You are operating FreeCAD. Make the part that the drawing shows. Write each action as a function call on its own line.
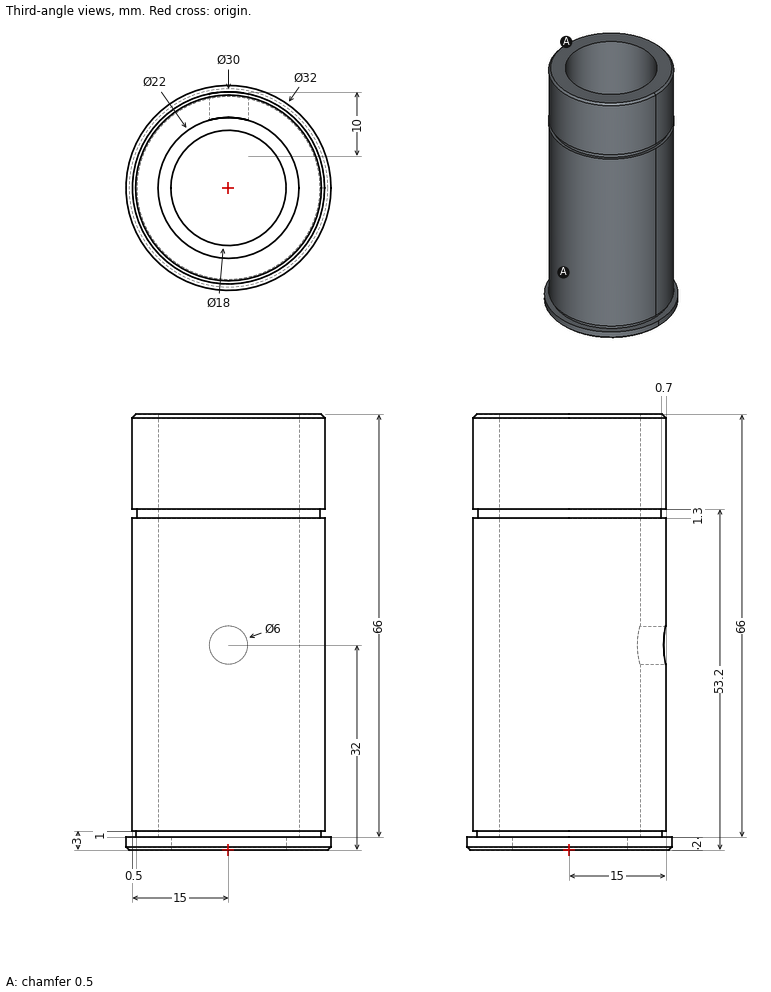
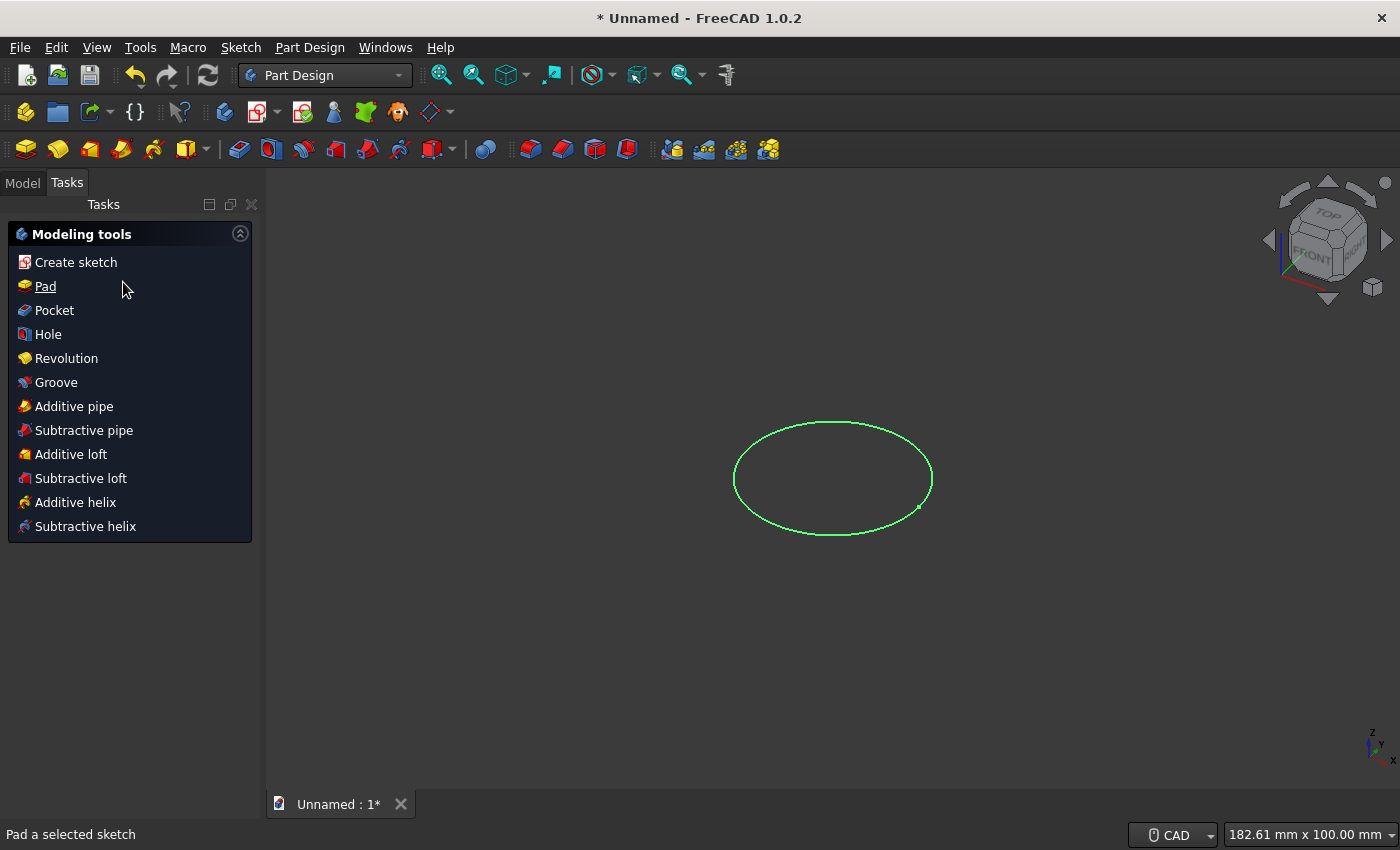
click(26, 150)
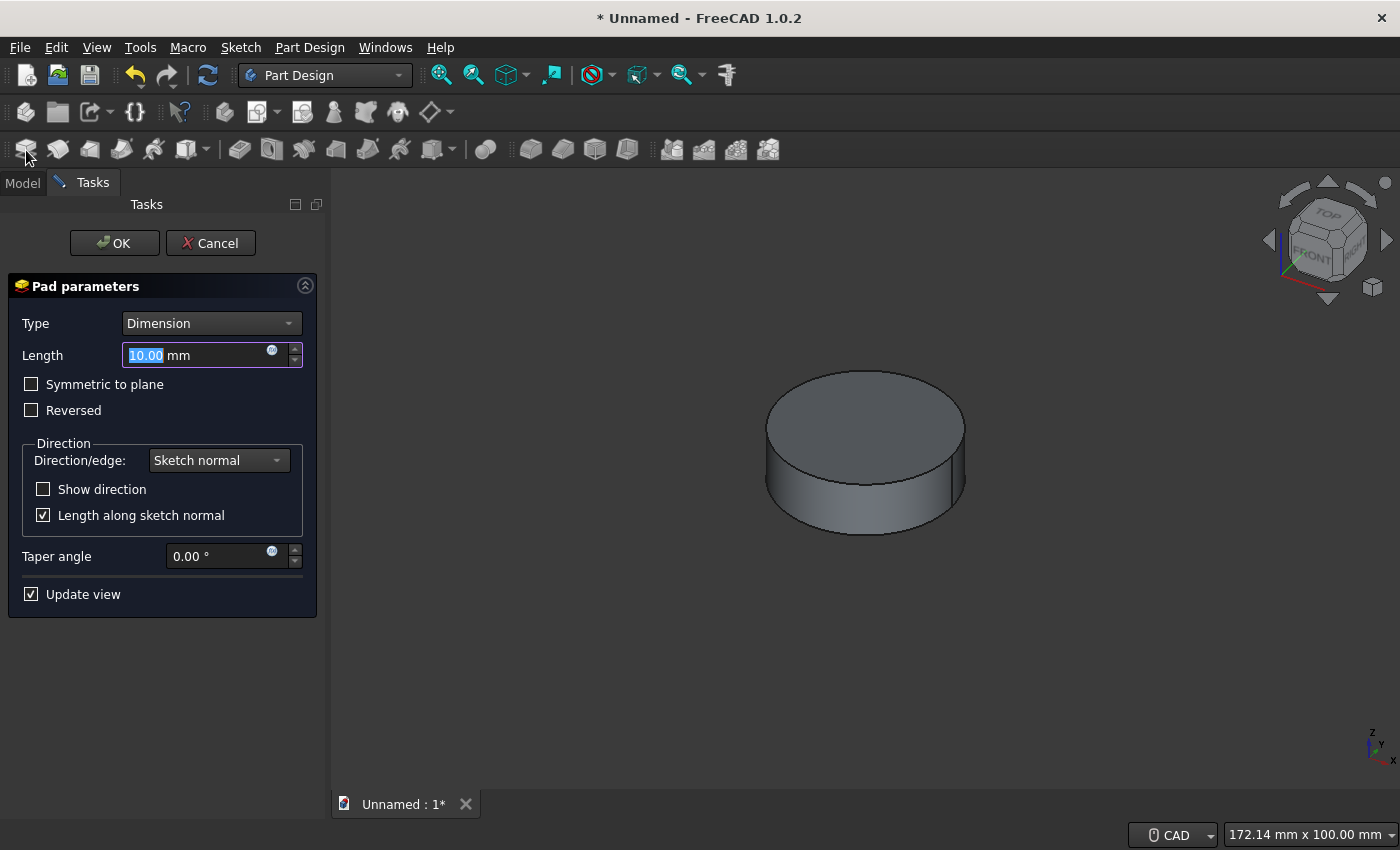
text(2)
key(Tab)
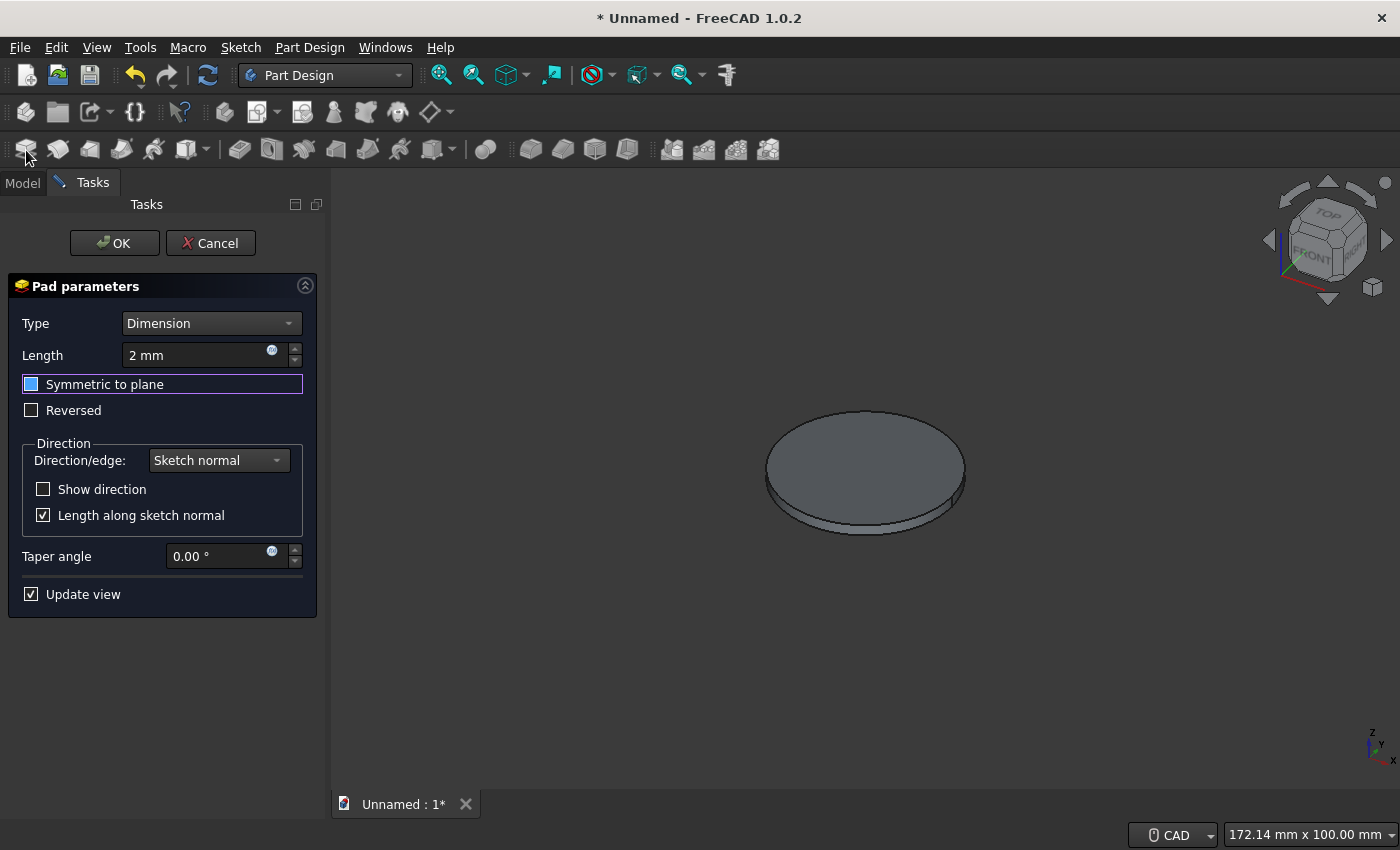
click(115, 243)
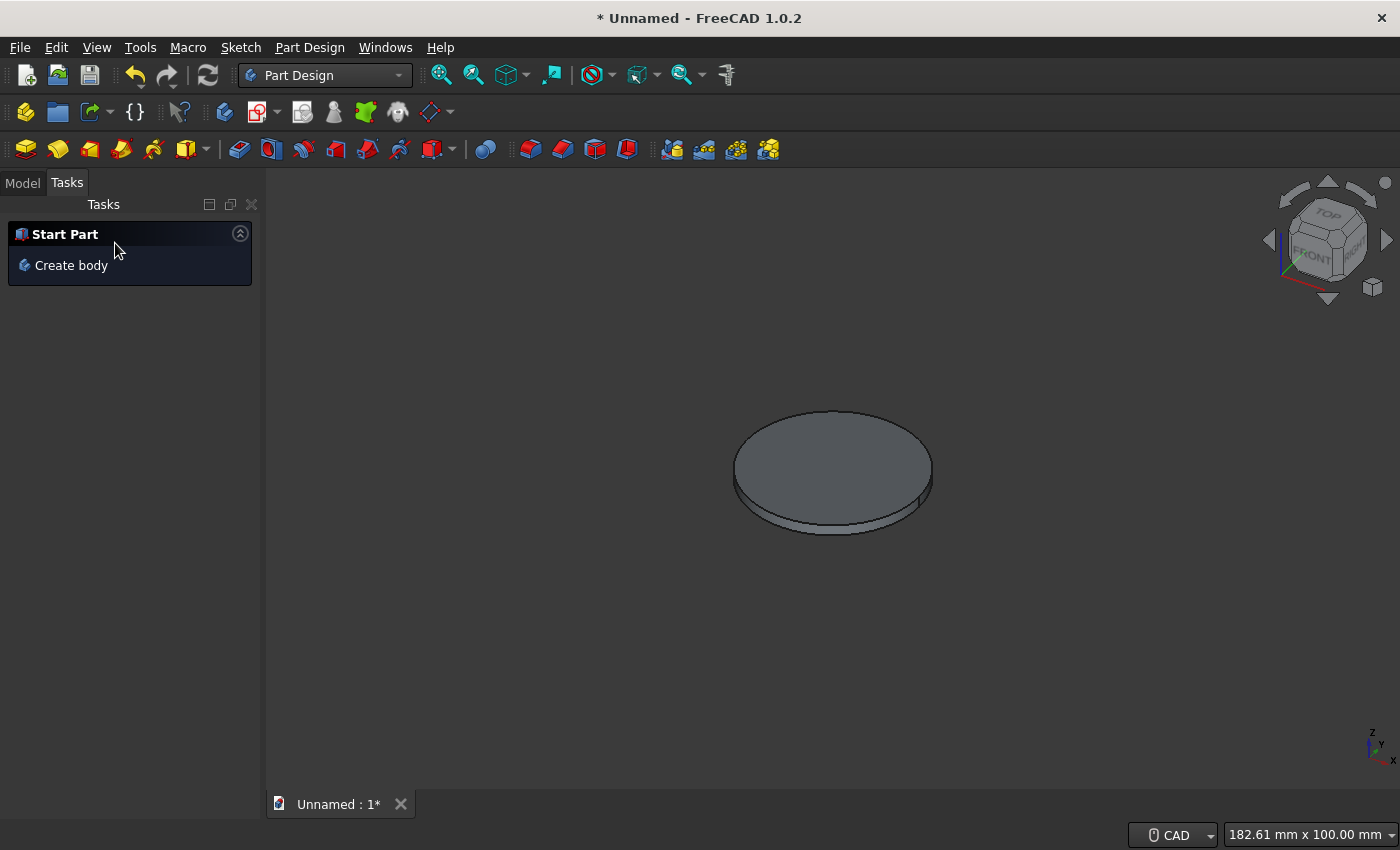
click(442, 76)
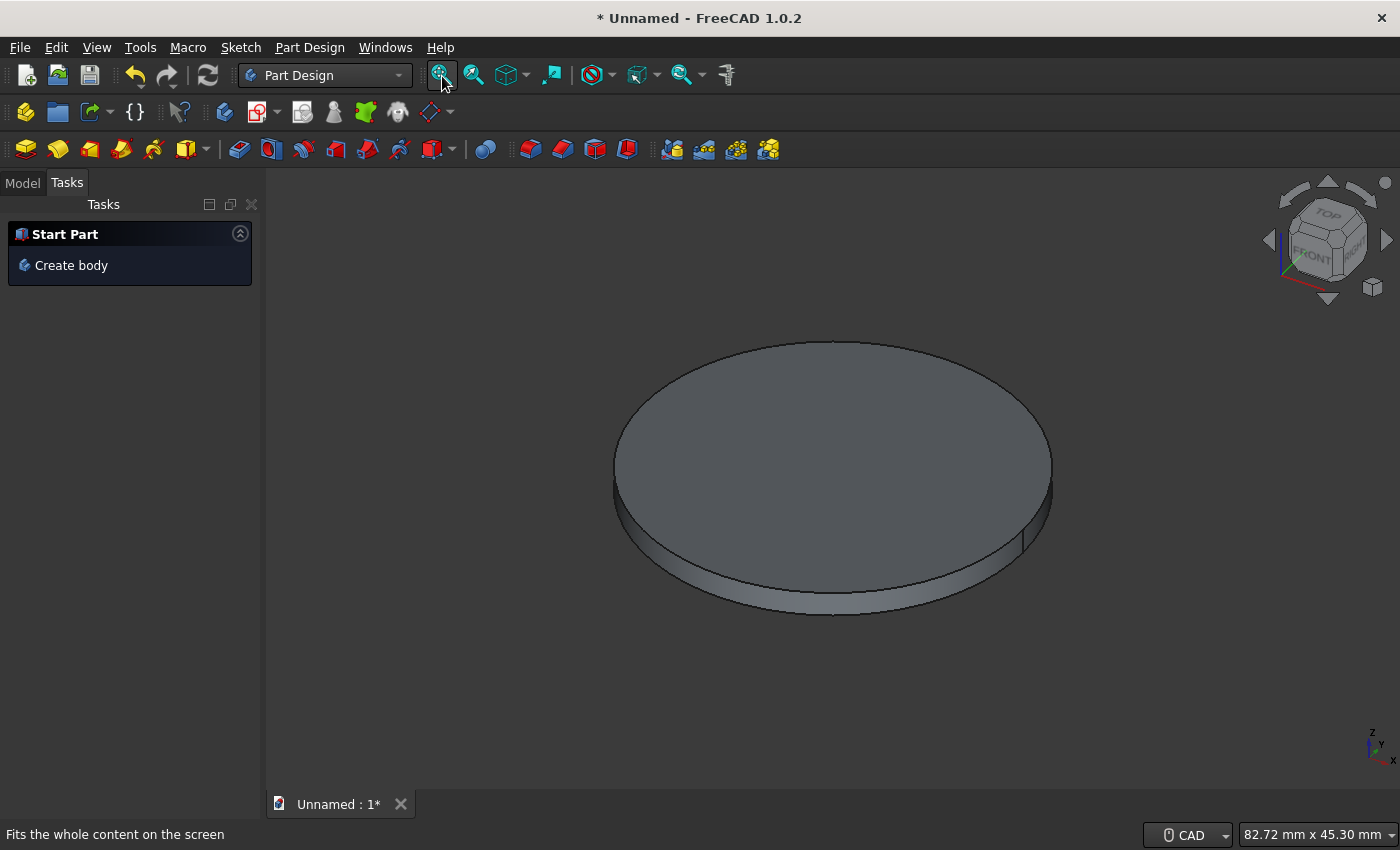
click(833, 466)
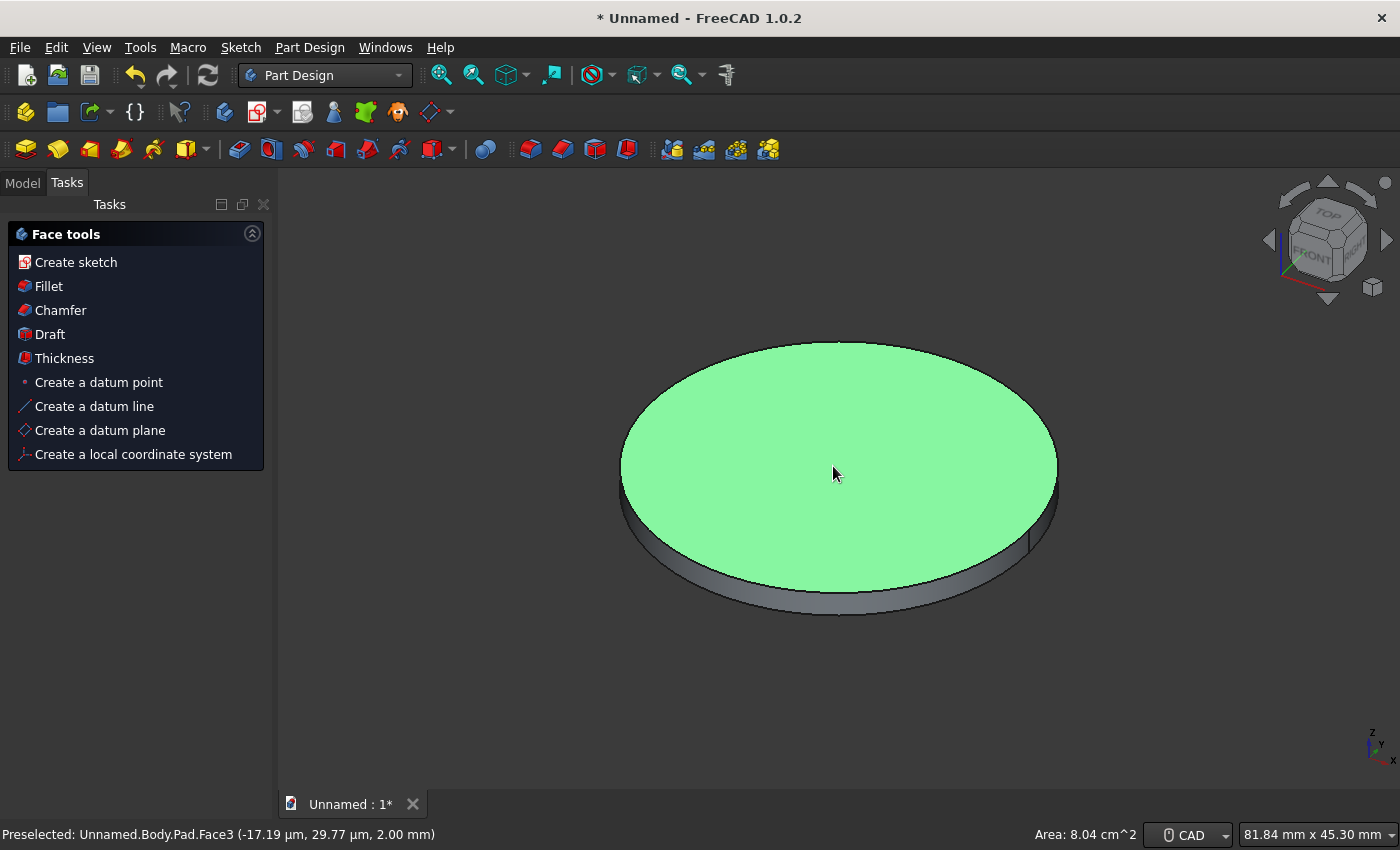
click(258, 112)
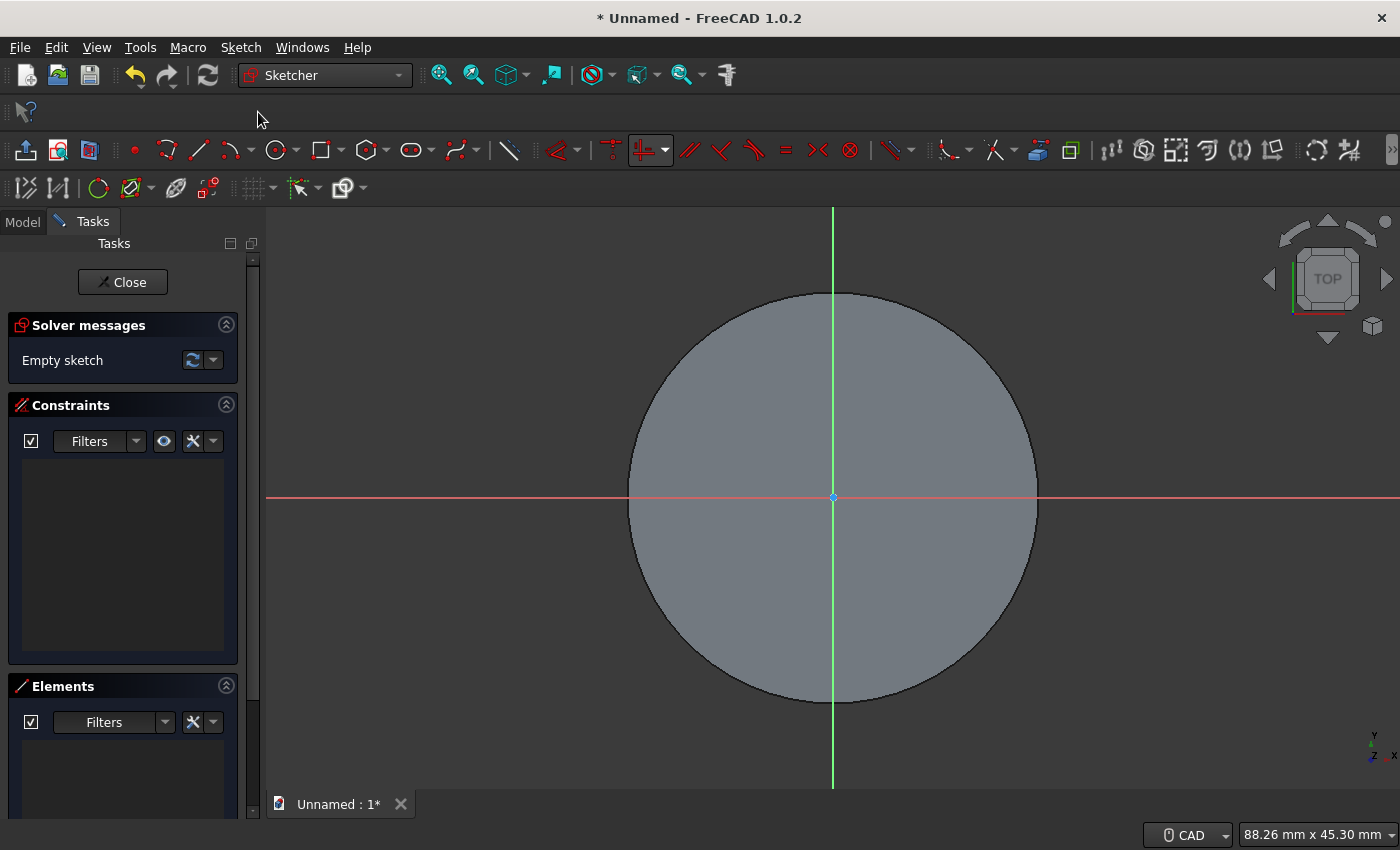
click(276, 150)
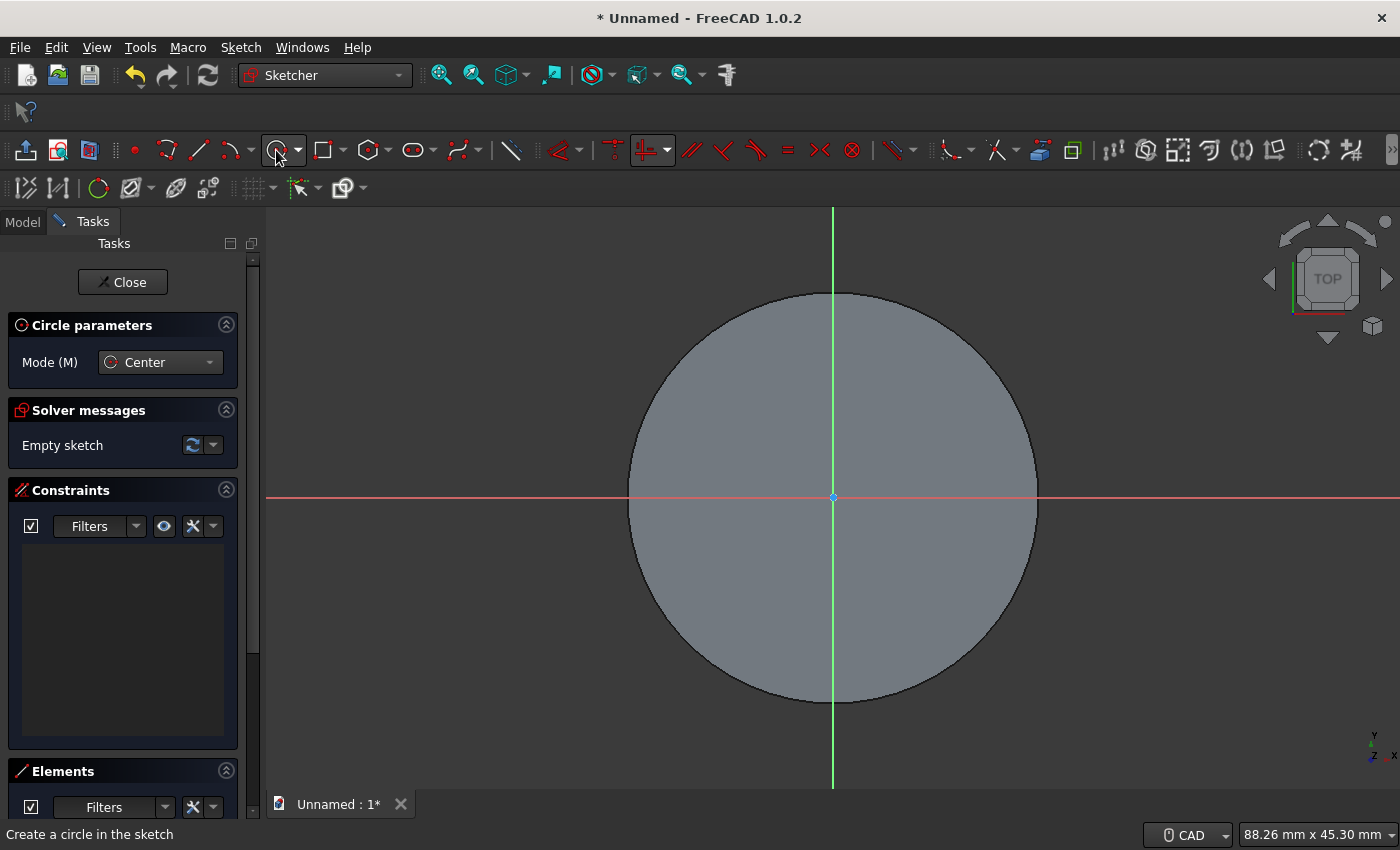
click(833, 498)
move(969, 362)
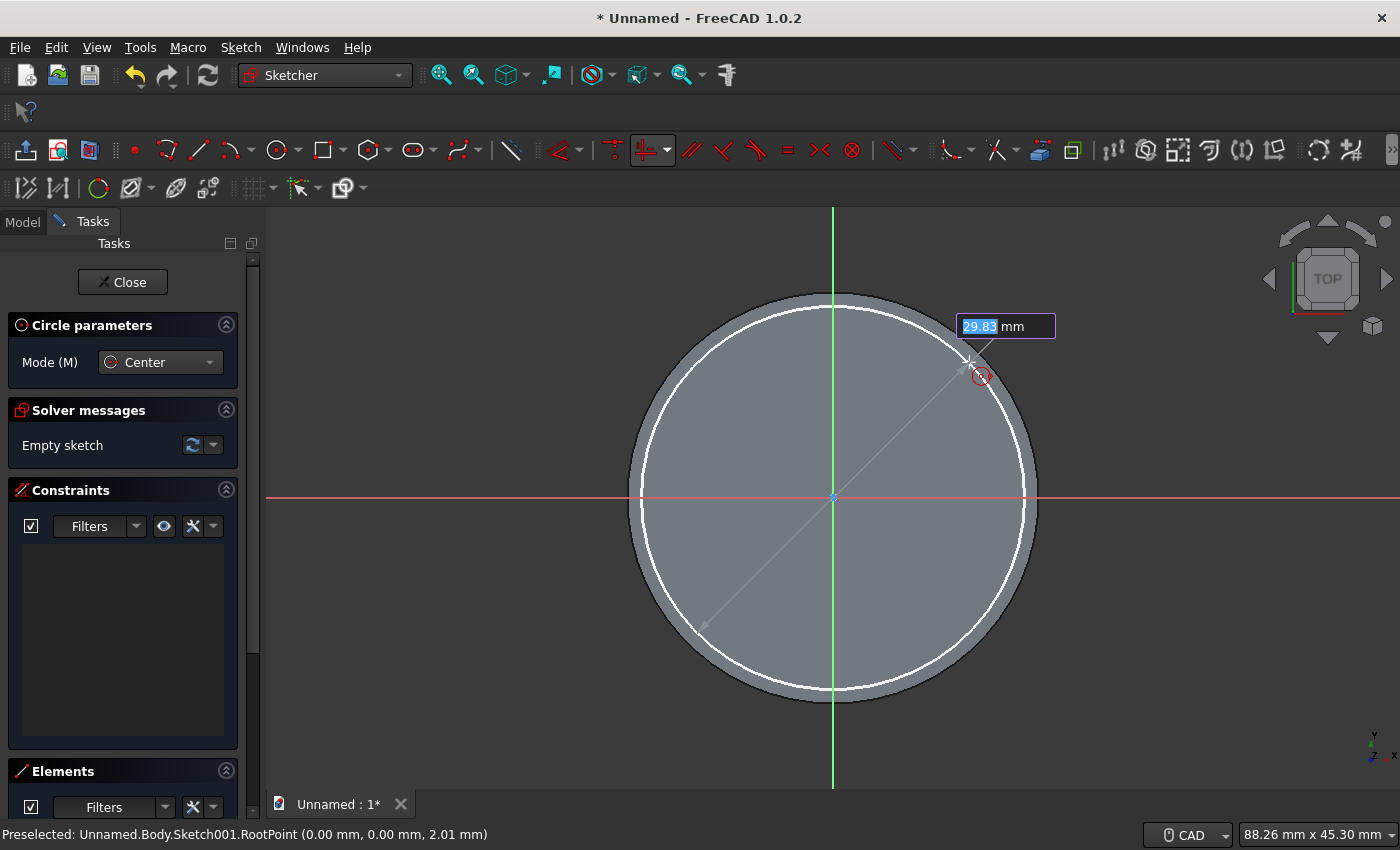
text(30)
key(Return)
key(Escape)